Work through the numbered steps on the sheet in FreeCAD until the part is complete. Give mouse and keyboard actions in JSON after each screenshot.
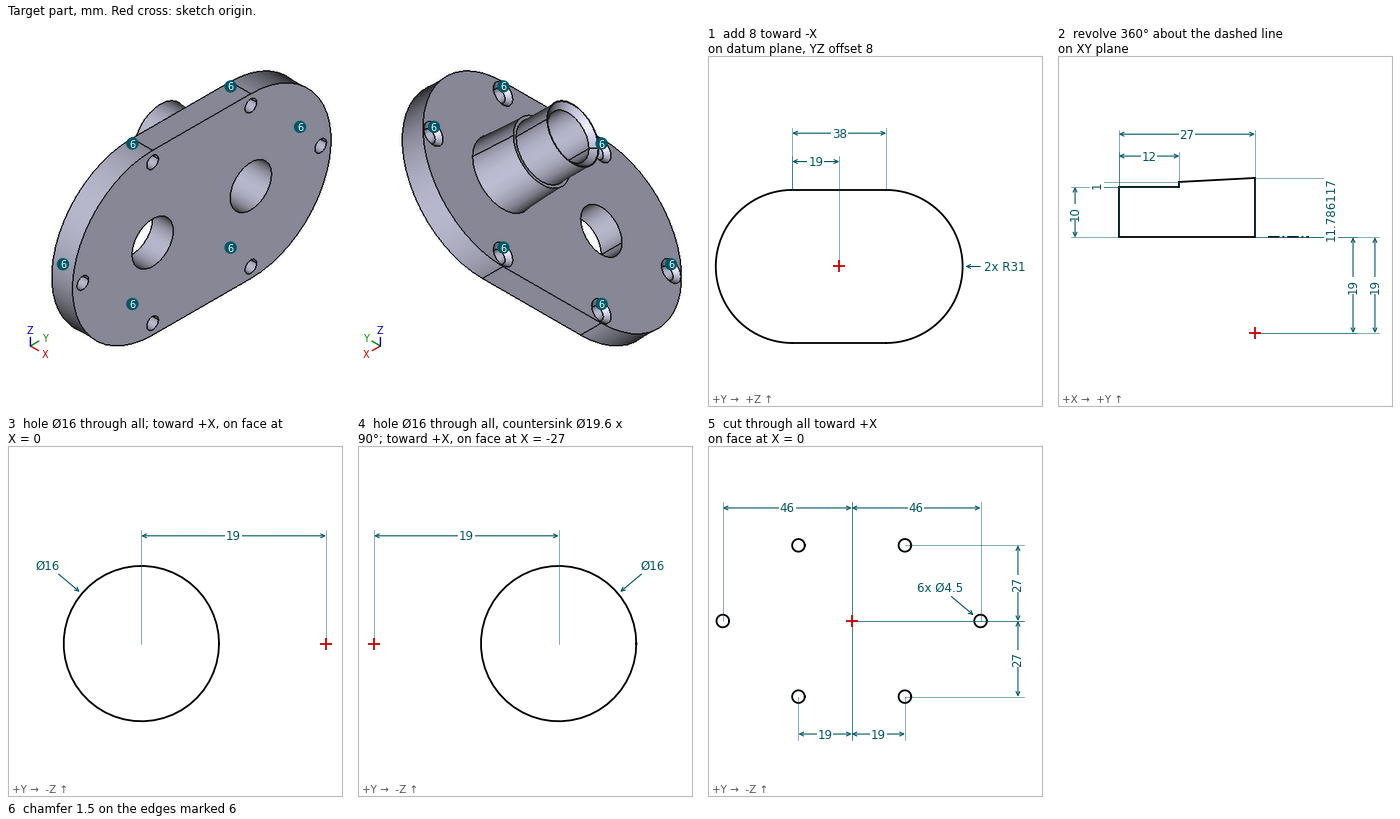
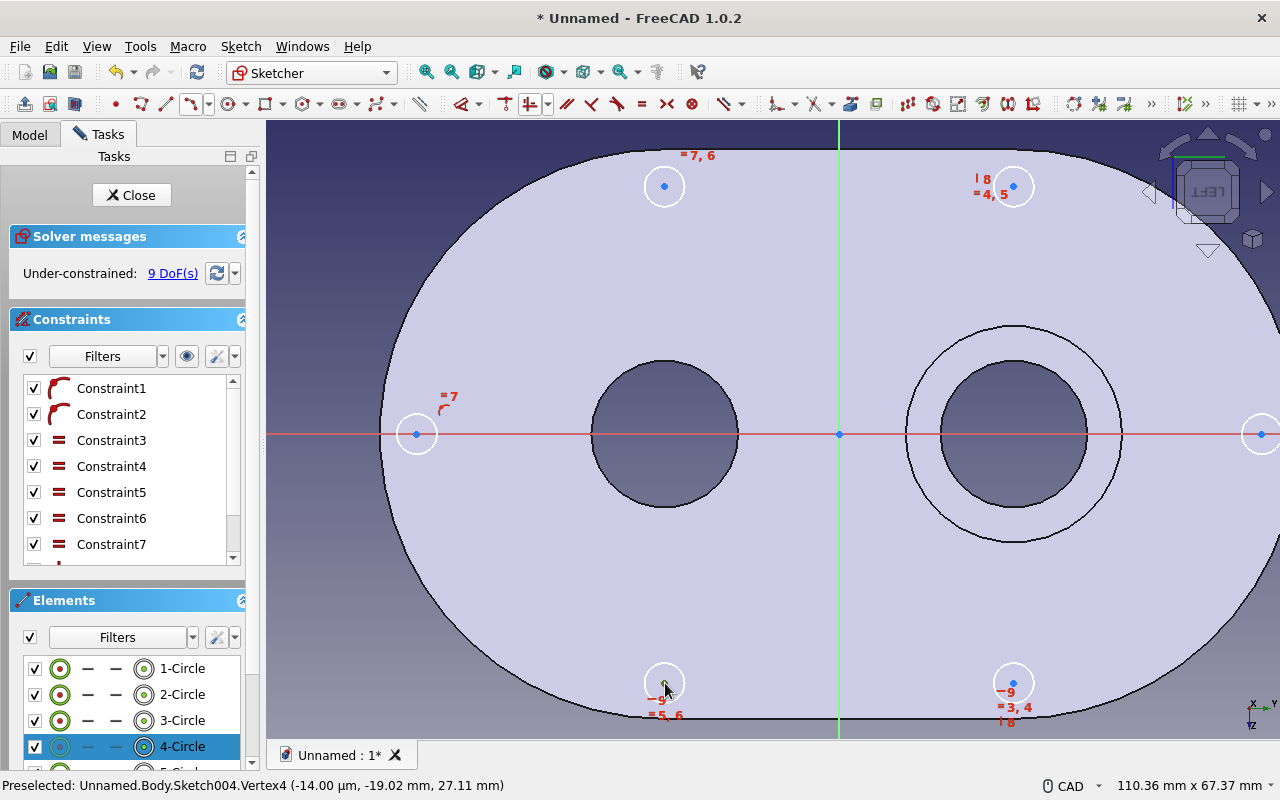
{"action": "left_click", "coordinate": [665, 187]}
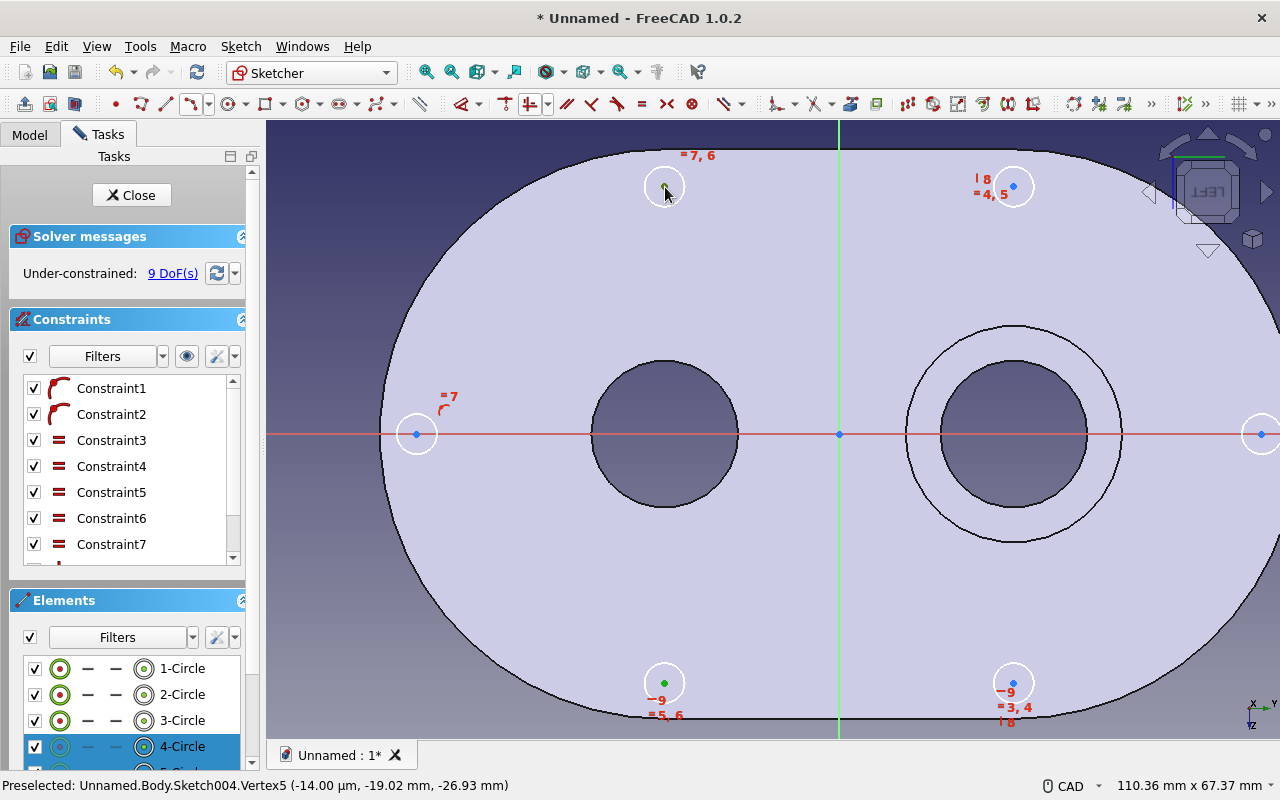
{"action": "key", "text": "v"}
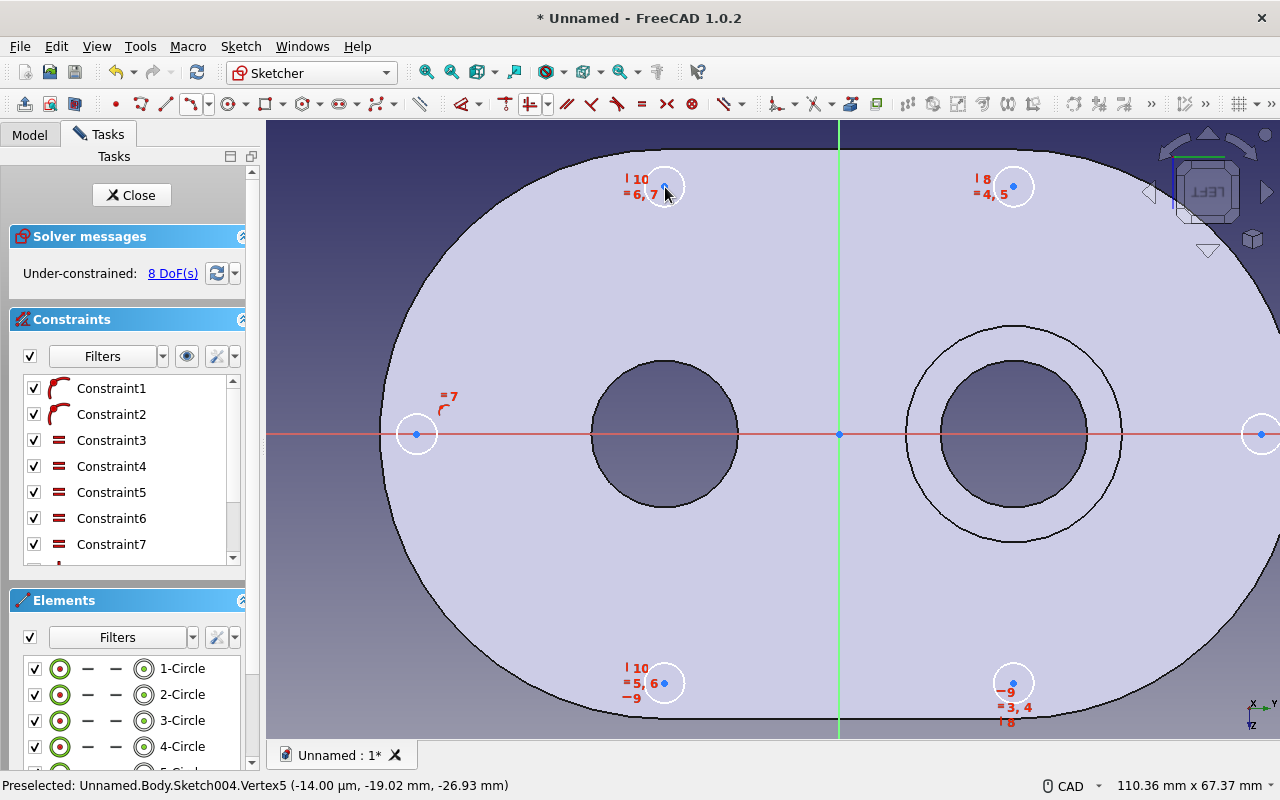
{"action": "left_click", "coordinate": [1014, 187]}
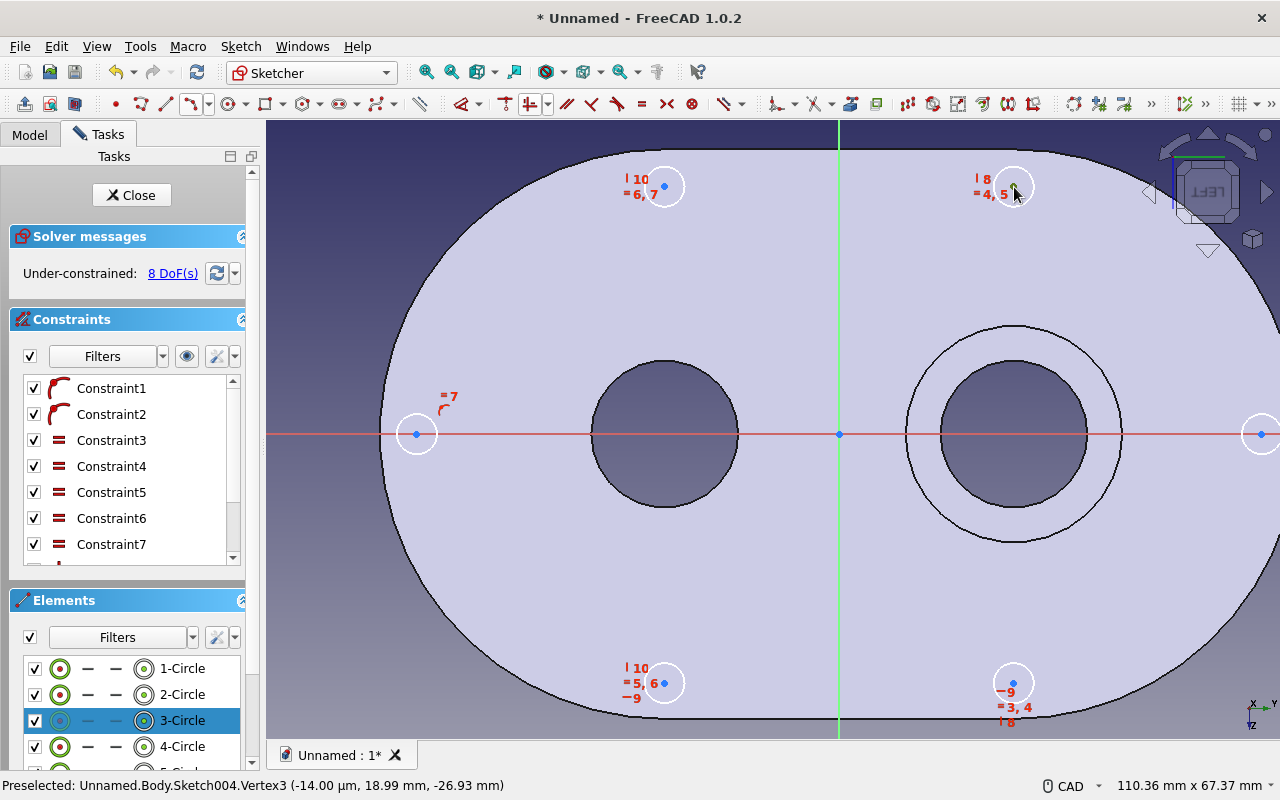
{"action": "left_click", "coordinate": [665, 187]}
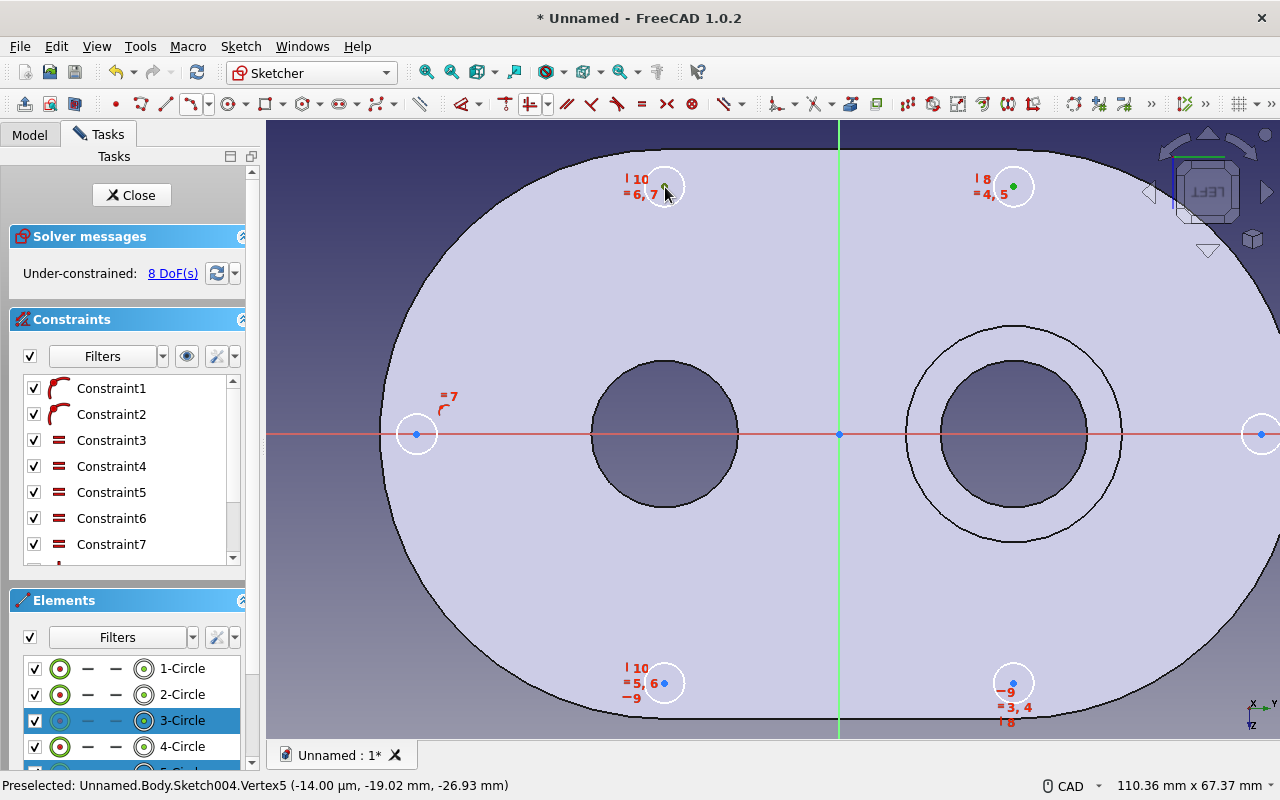
{"action": "key", "text": "h"}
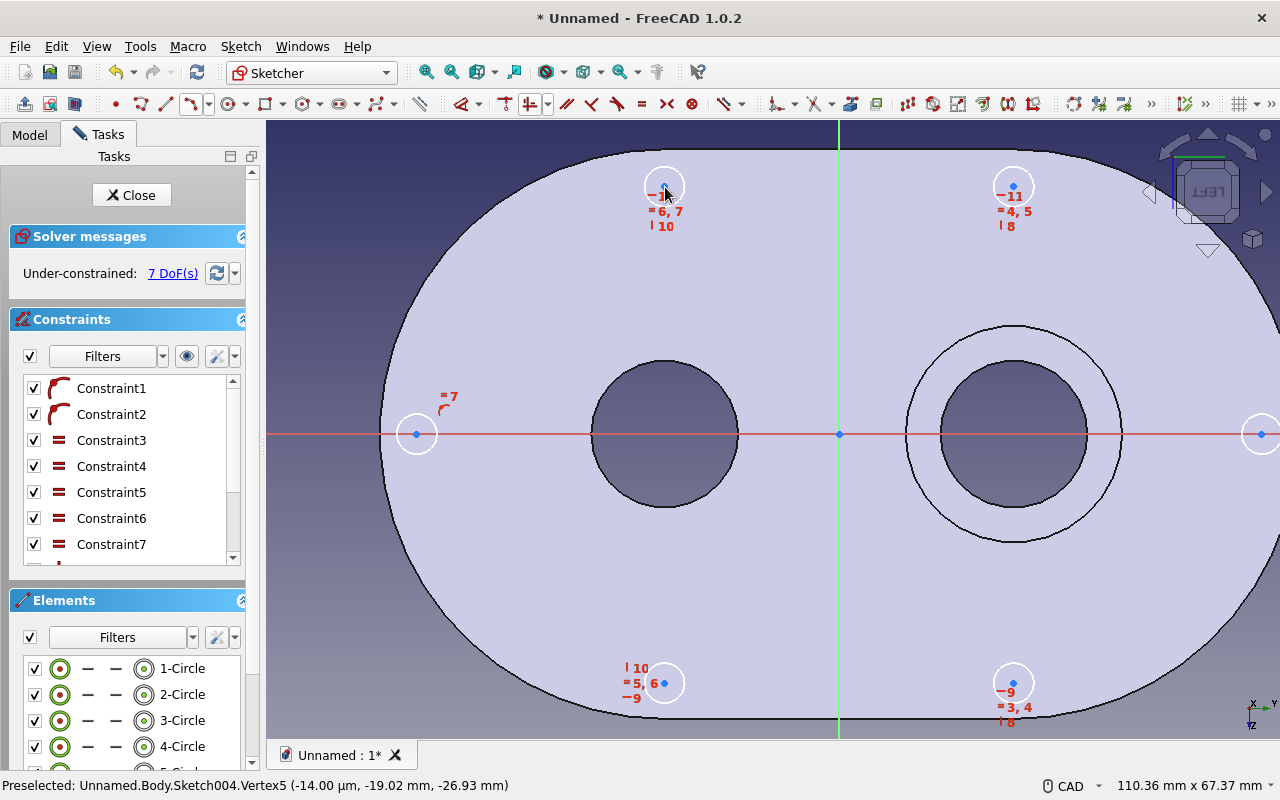
{"action": "key", "text": "d"}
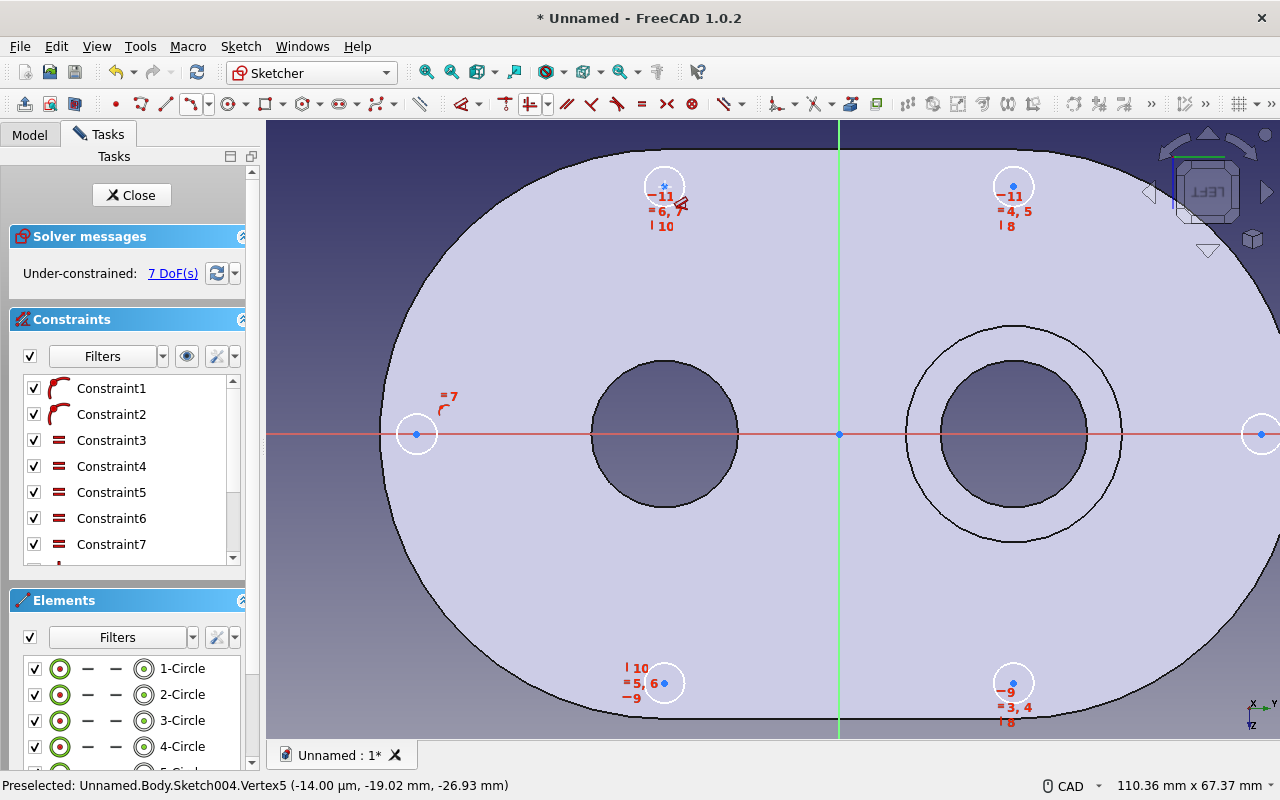
{"action": "scroll", "coordinate": [430, 420], "scroll_direction": "down", "scroll_amount": 2}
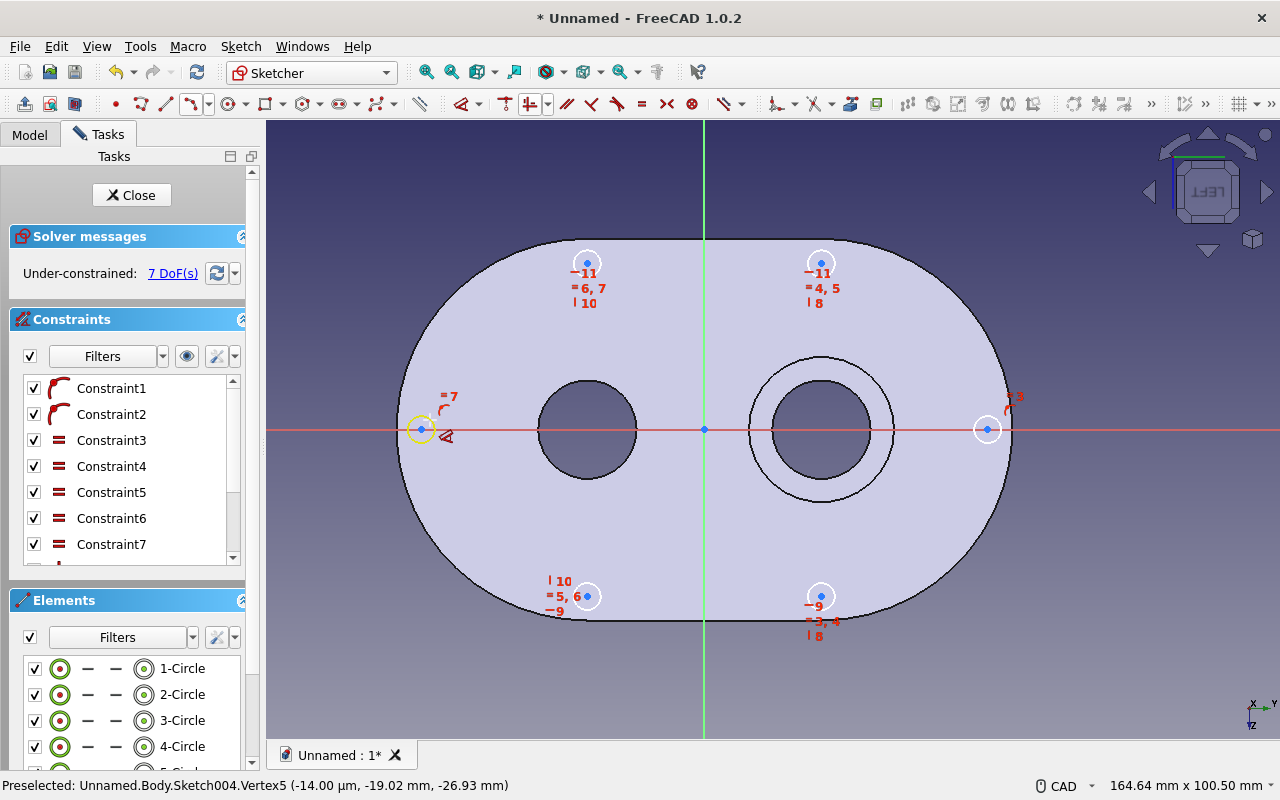
{"action": "scroll", "coordinate": [997, 420], "scroll_direction": "up", "scroll_amount": 2}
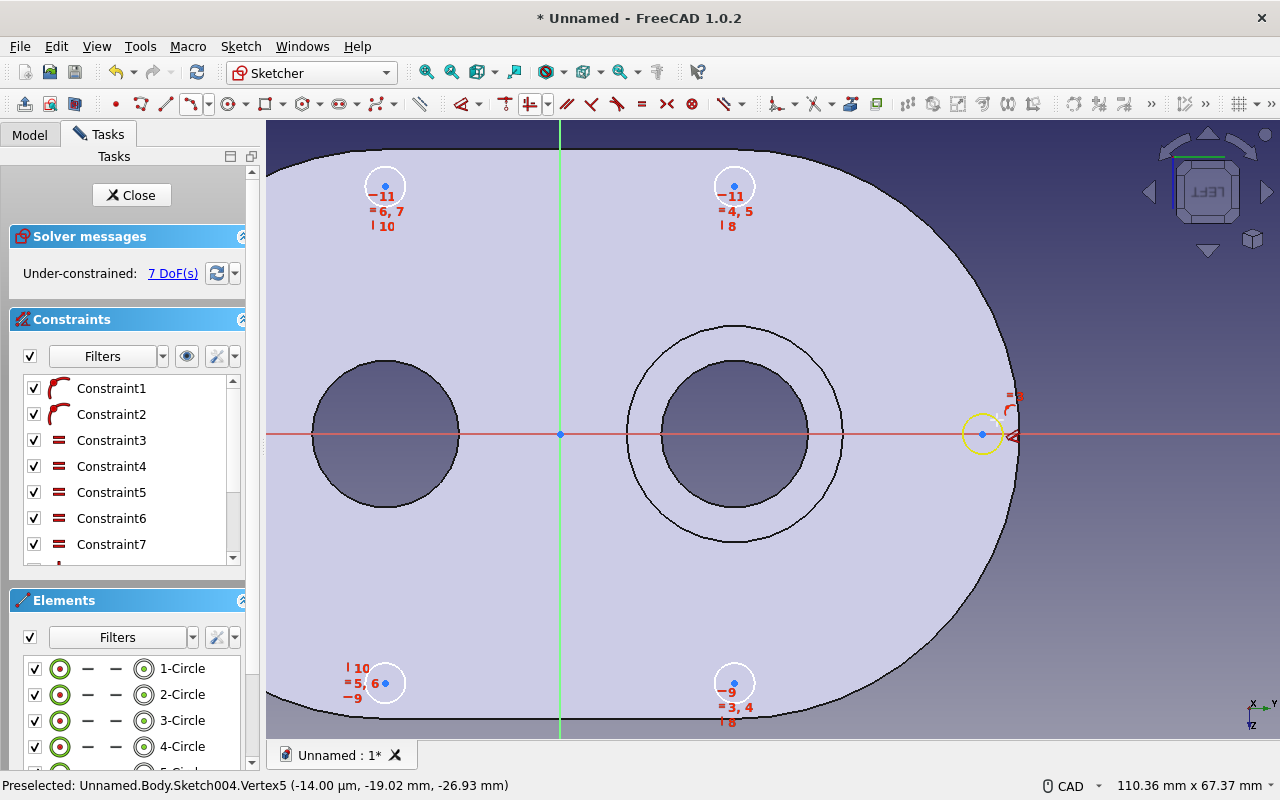
{"action": "left_click", "coordinate": [997, 420]}
{"action": "left_click", "coordinate": [1020, 397]}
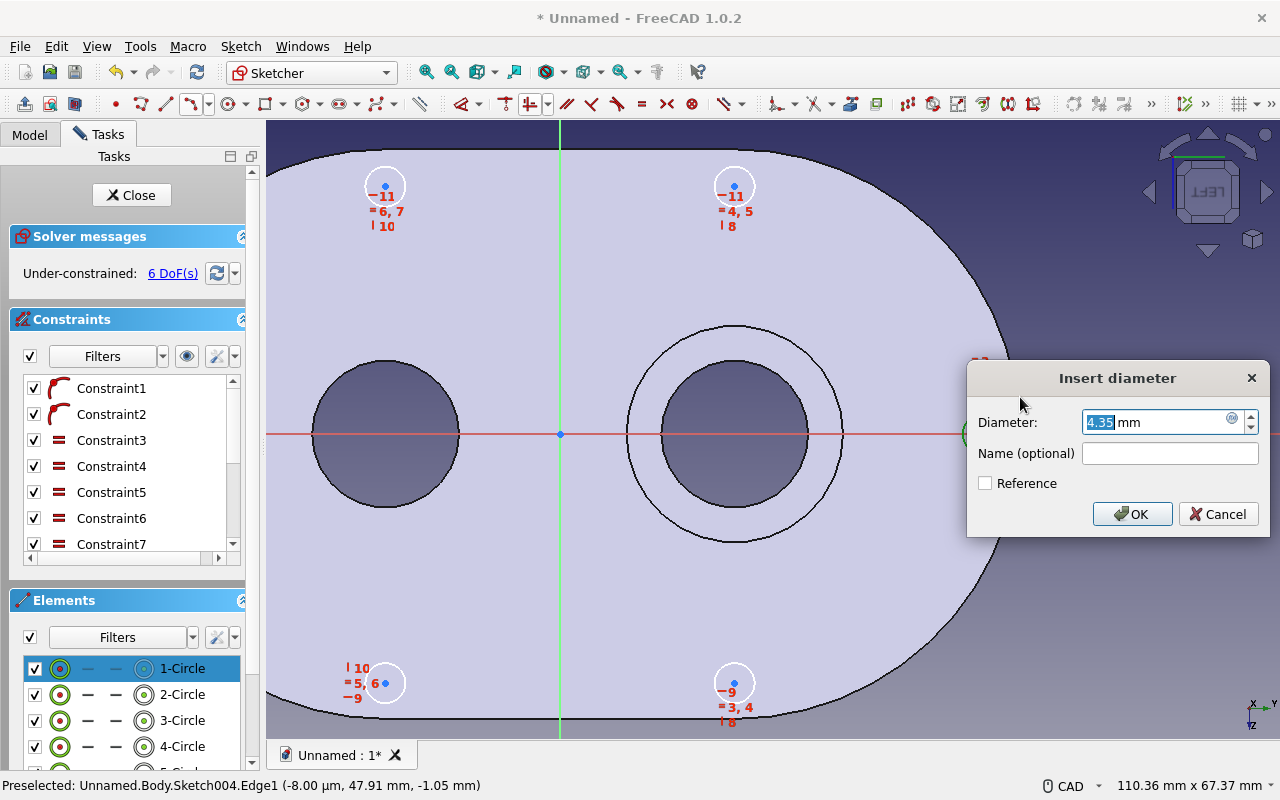
{"action": "type", "text": "4.5"}
{"action": "key", "text": "Return"}